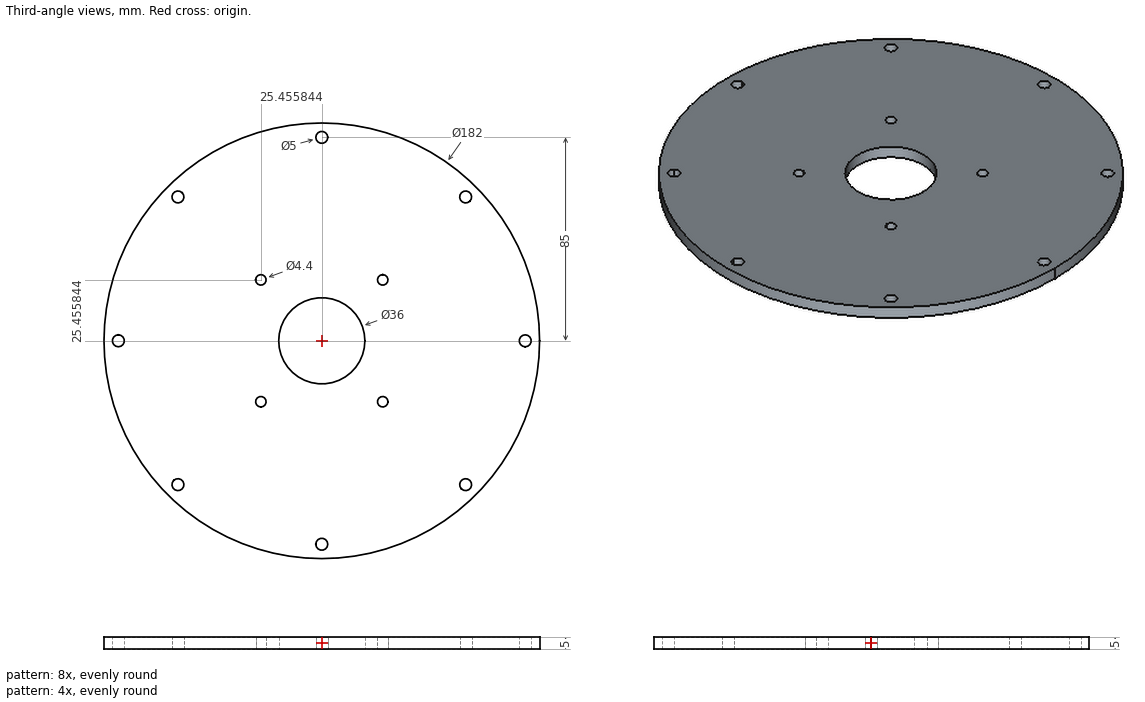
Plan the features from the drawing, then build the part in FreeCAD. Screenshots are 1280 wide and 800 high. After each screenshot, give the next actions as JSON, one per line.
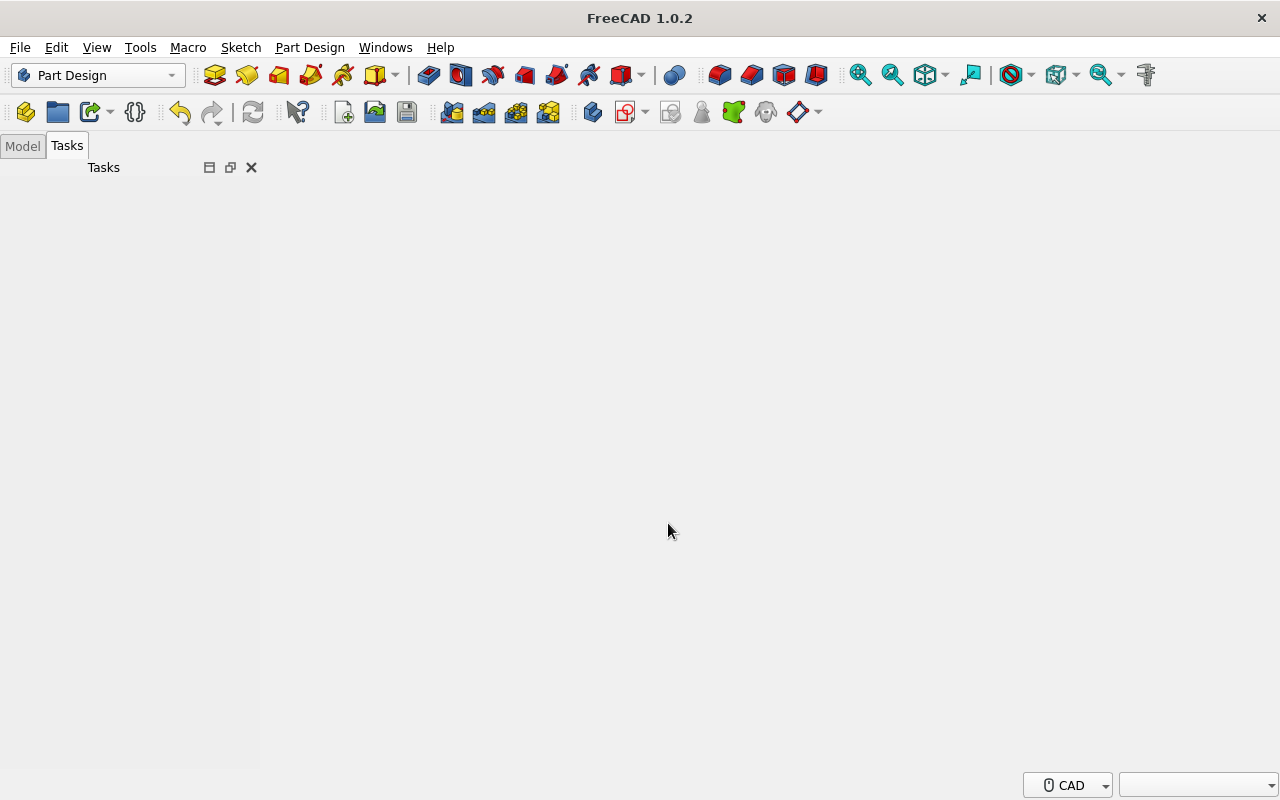
{"action": "left_click", "coordinate": [344, 112]}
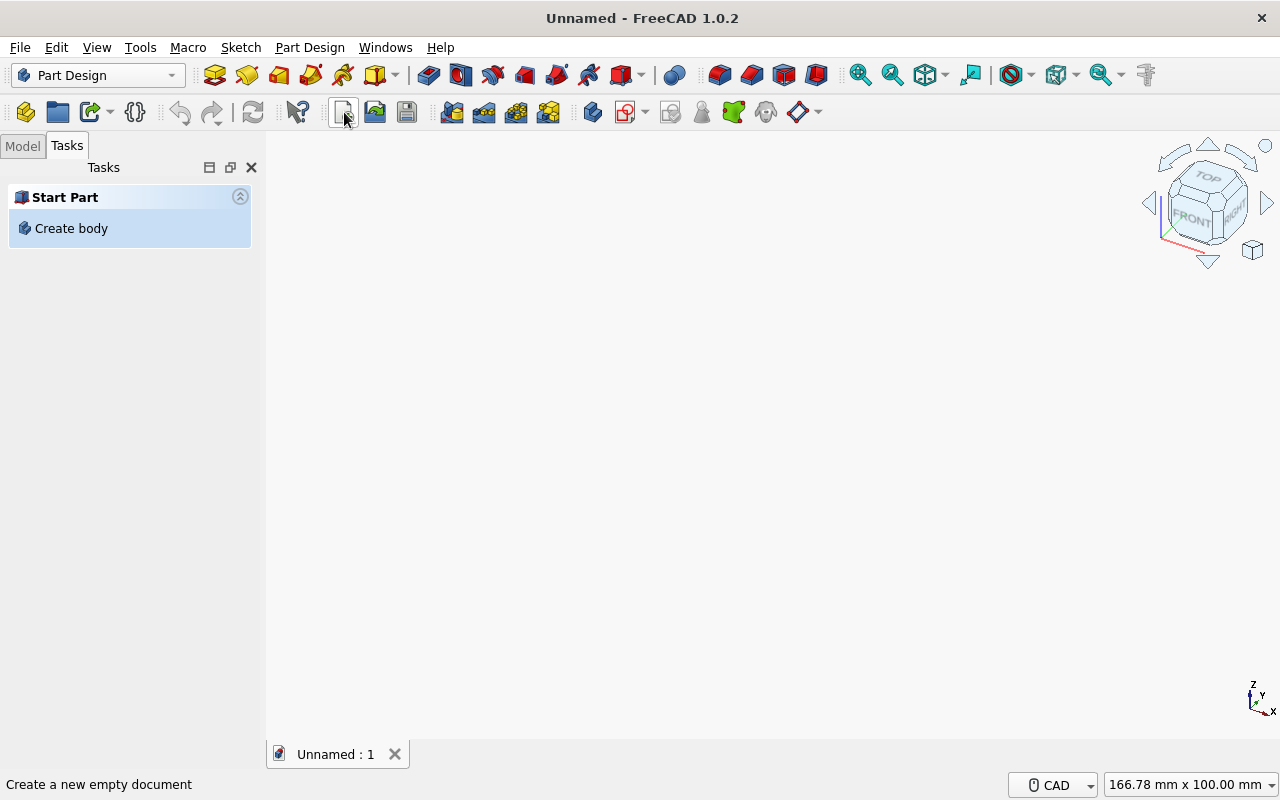
{"action": "left_click", "coordinate": [626, 112]}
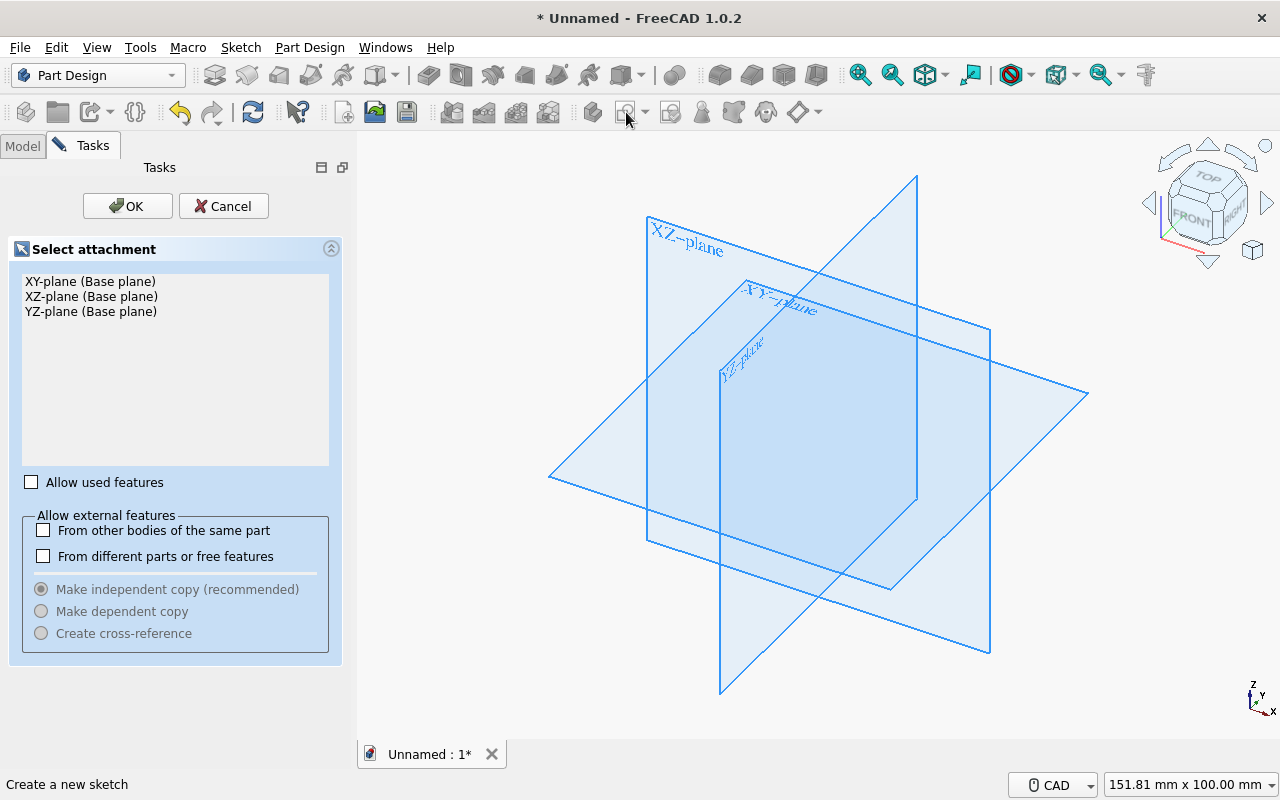
{"action": "left_click", "coordinate": [82, 282]}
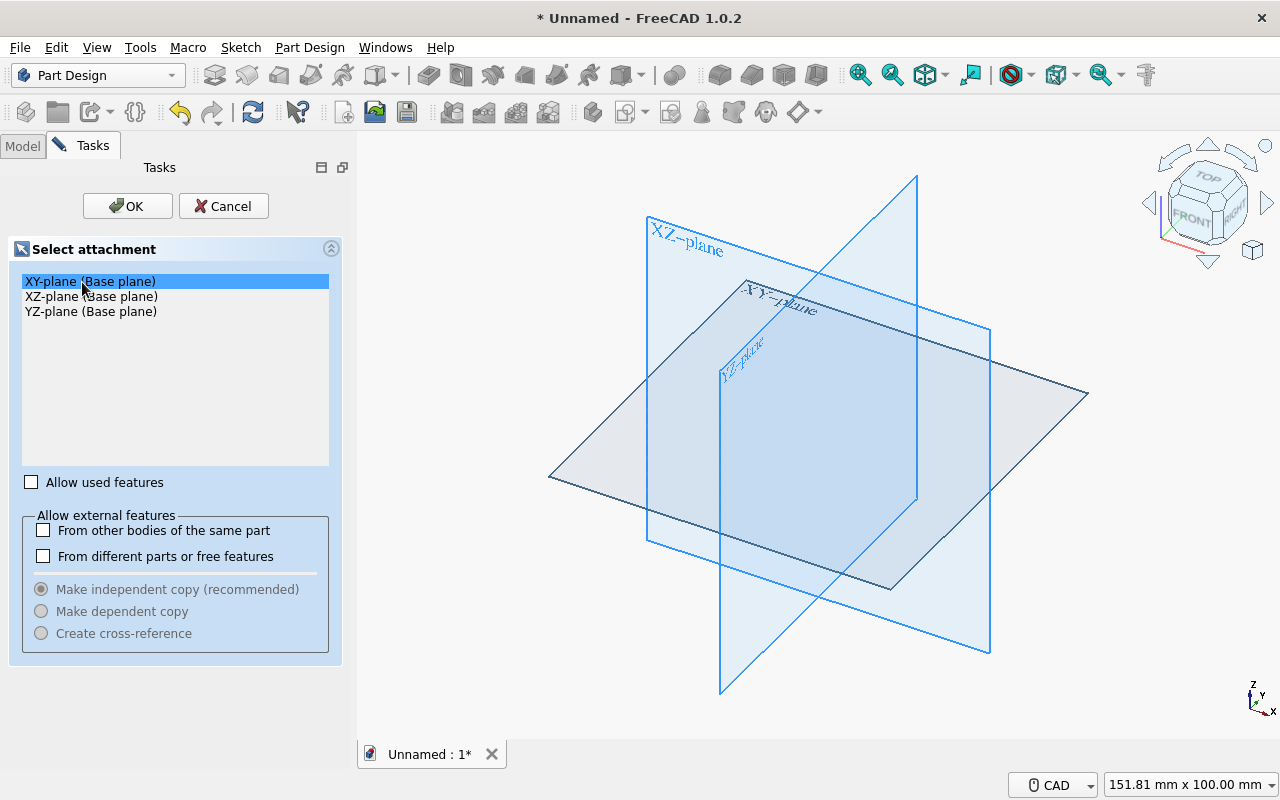
{"action": "left_click", "coordinate": [128, 206]}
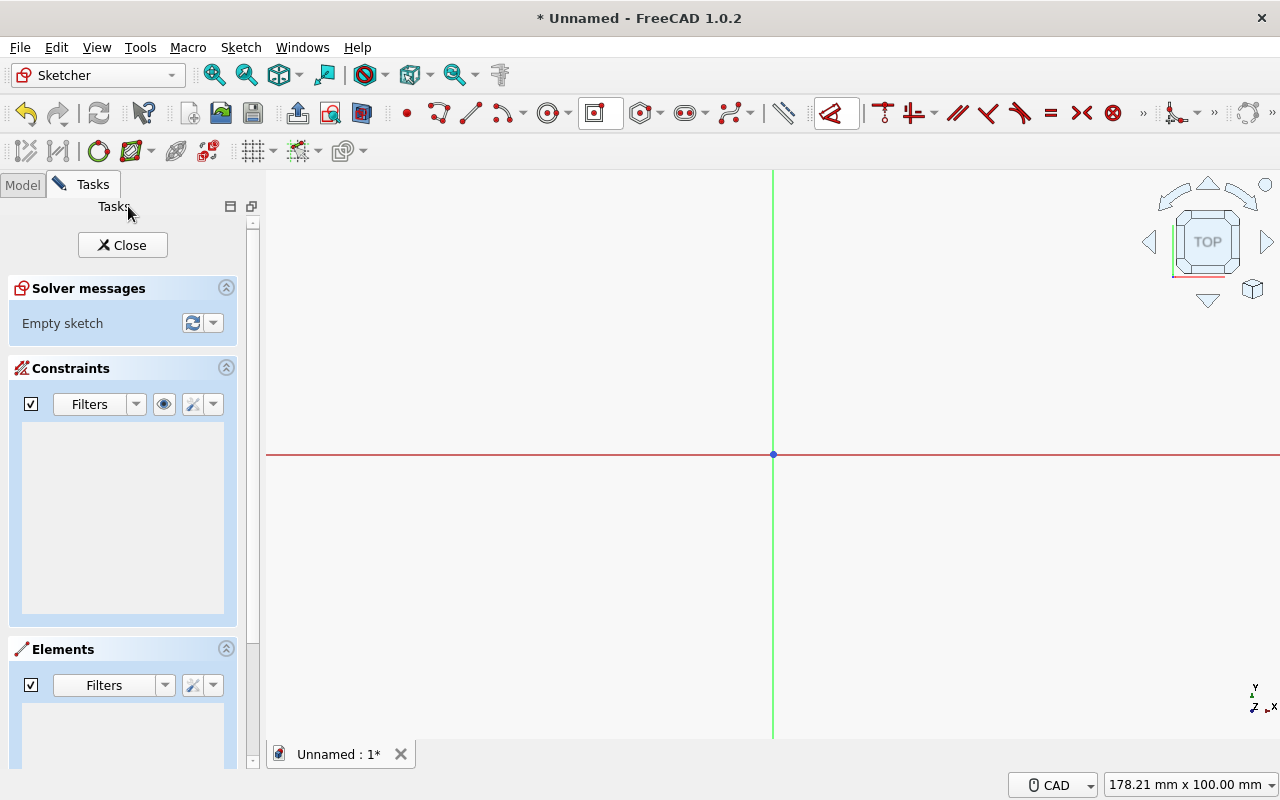
{"action": "scroll", "coordinate": [665, 454], "scroll_direction": "down", "scroll_amount": 5}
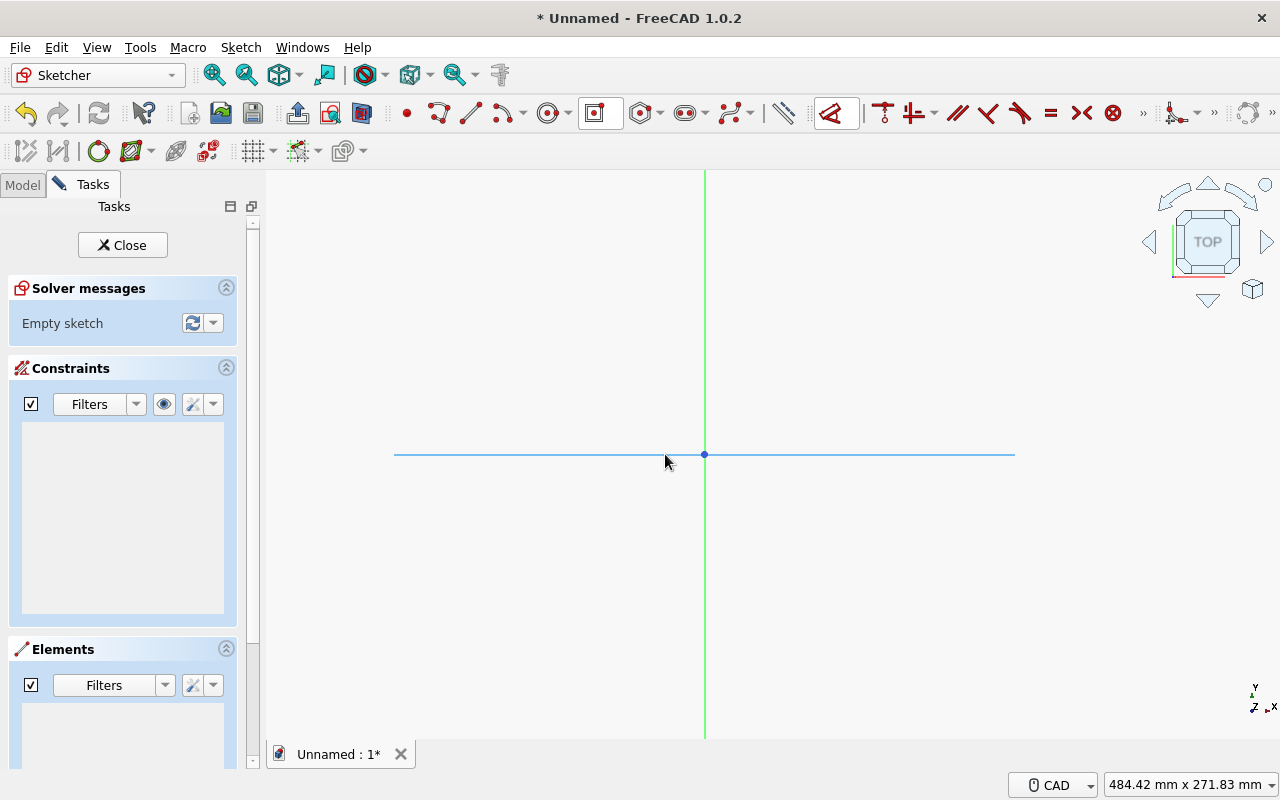
{"action": "left_click", "coordinate": [548, 114]}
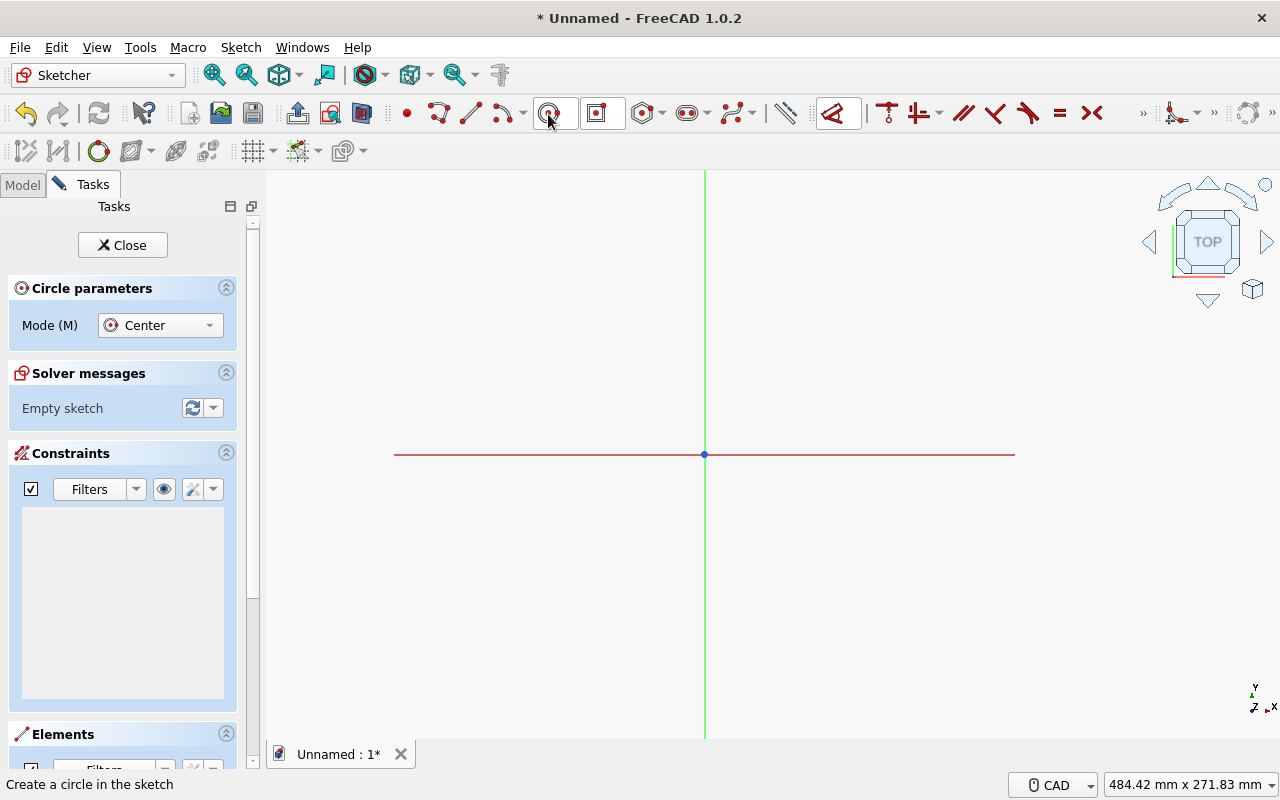
{"action": "left_click", "coordinate": [705, 454]}
{"action": "mouse_move", "coordinate": [840, 320]}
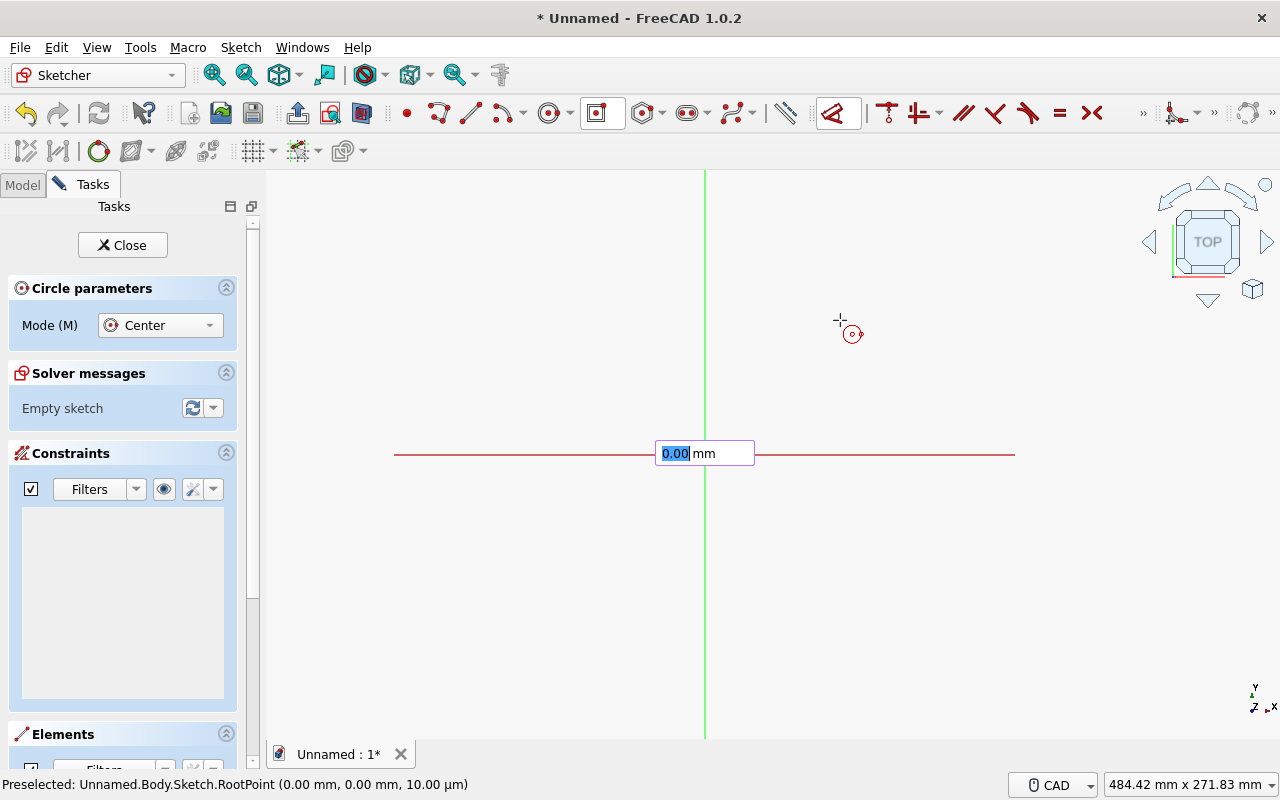
{"action": "type", "text": "182"}
{"action": "key", "text": "Return"}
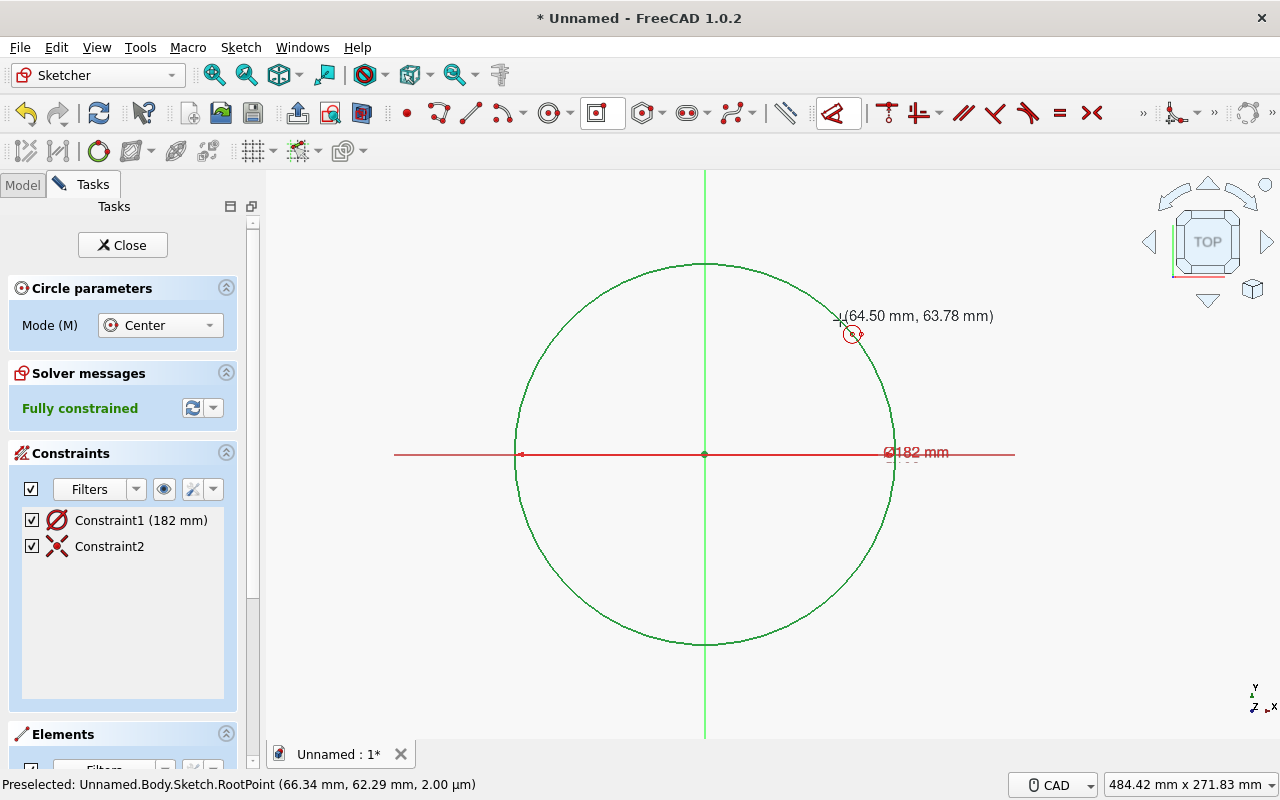
{"action": "left_click", "coordinate": [705, 454]}
{"action": "mouse_move", "coordinate": [732, 428]}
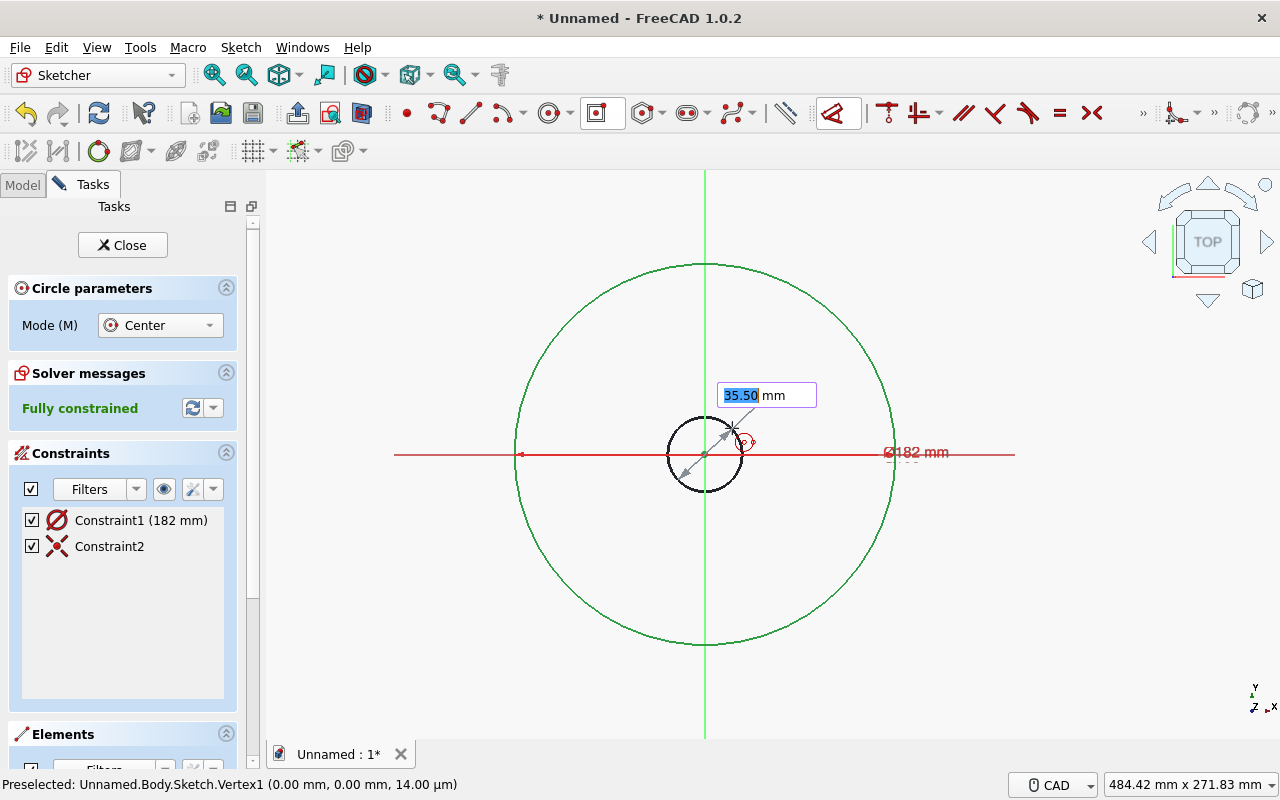
{"action": "type", "text": "36"}
{"action": "key", "text": "Return"}
{"action": "key", "text": "Escape"}